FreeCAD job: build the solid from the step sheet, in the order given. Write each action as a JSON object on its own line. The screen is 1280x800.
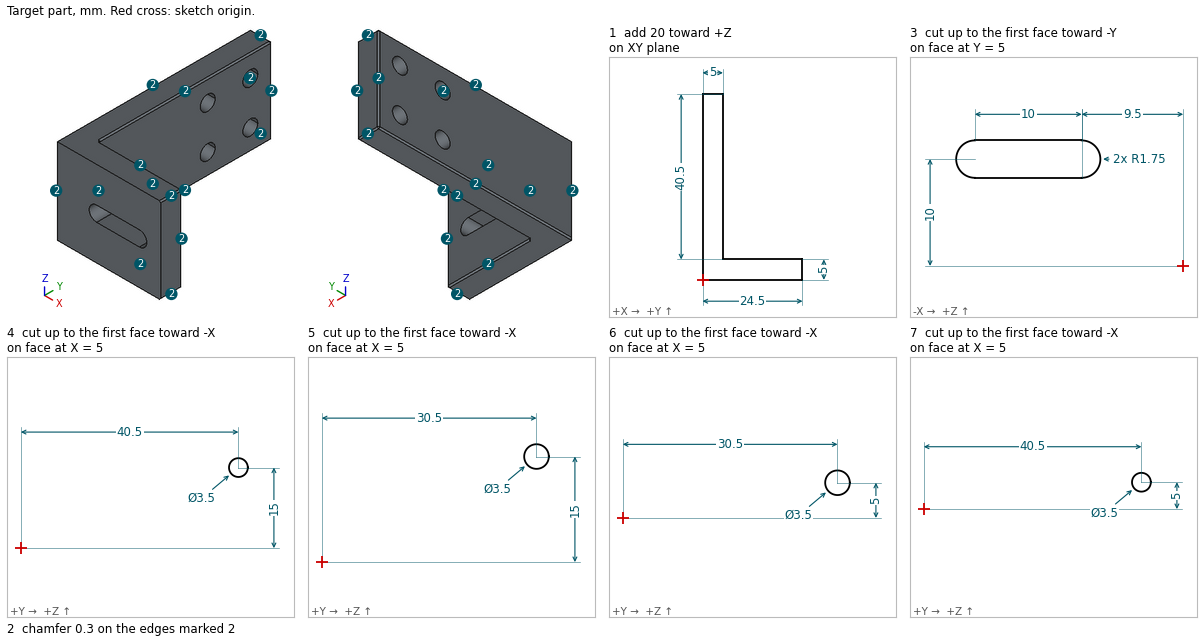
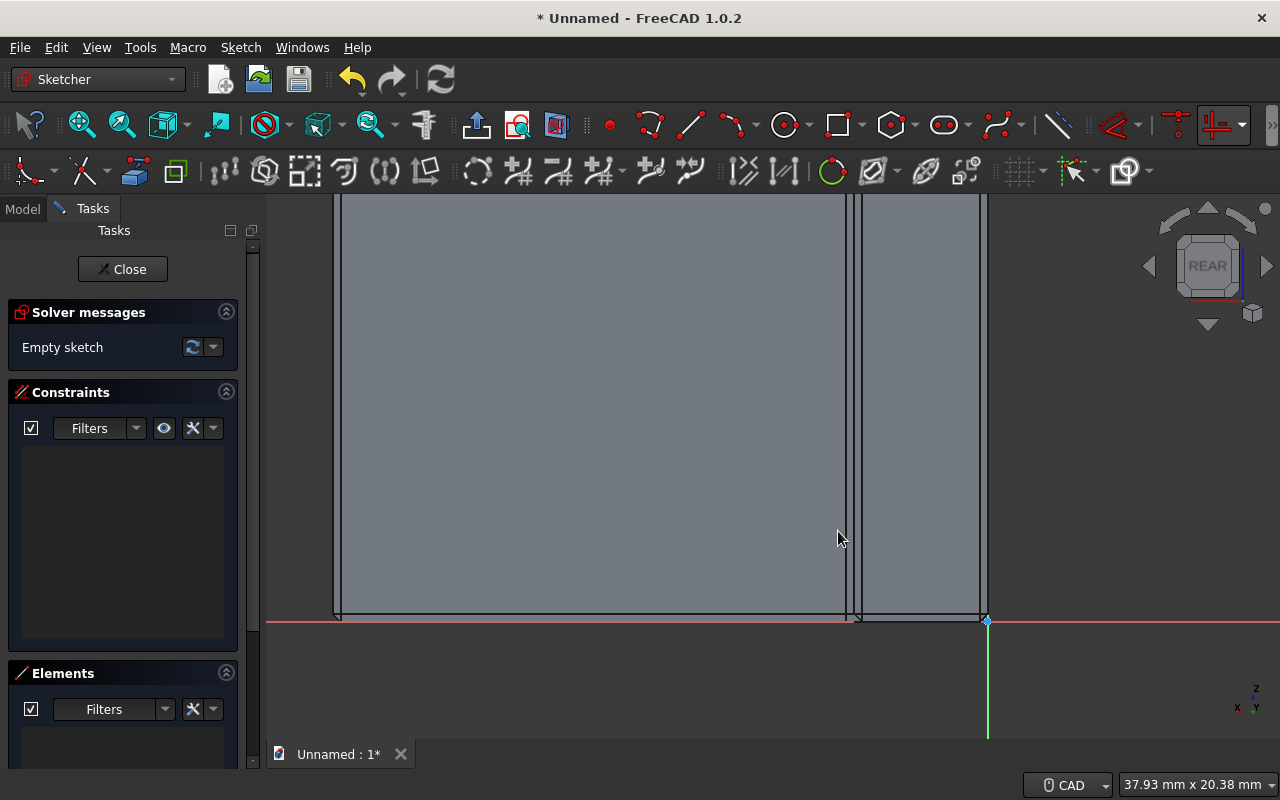
{"action": "left_click", "coordinate": [467, 355]}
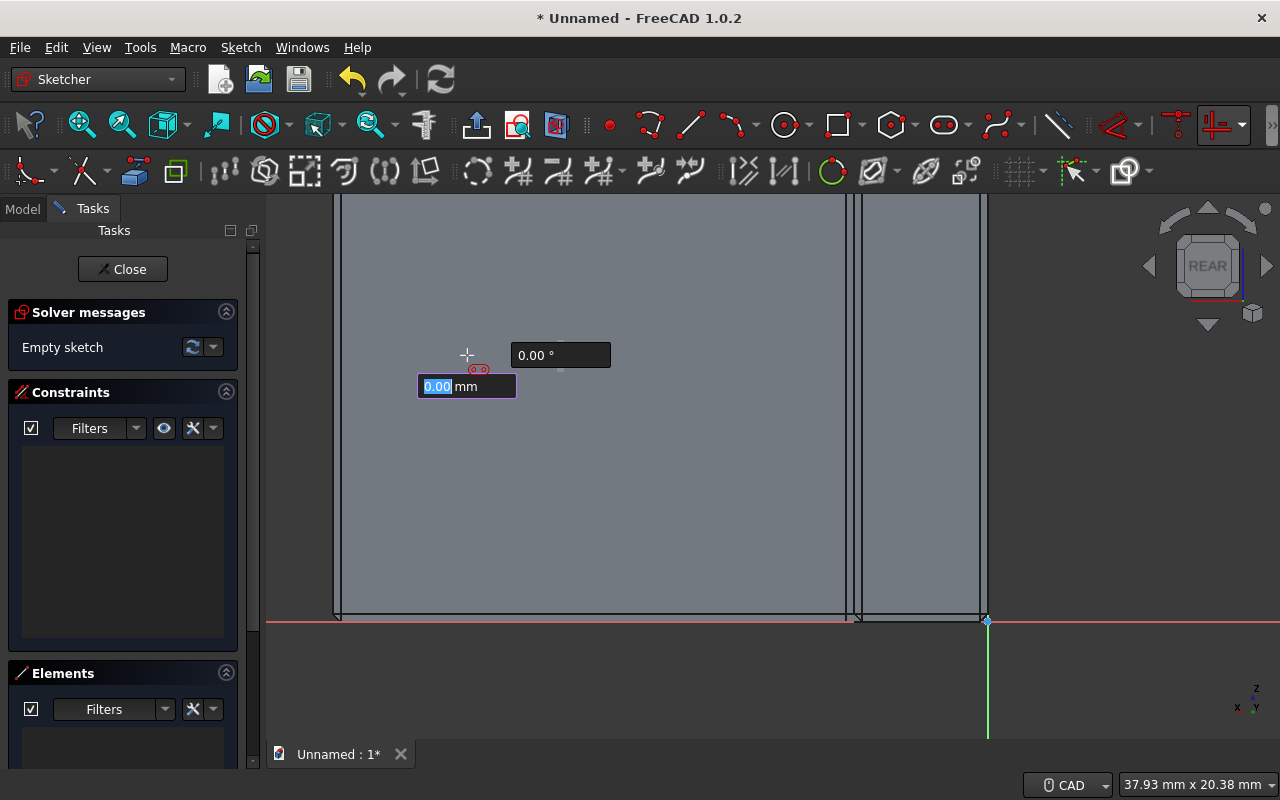
{"action": "left_click", "coordinate": [734, 355]}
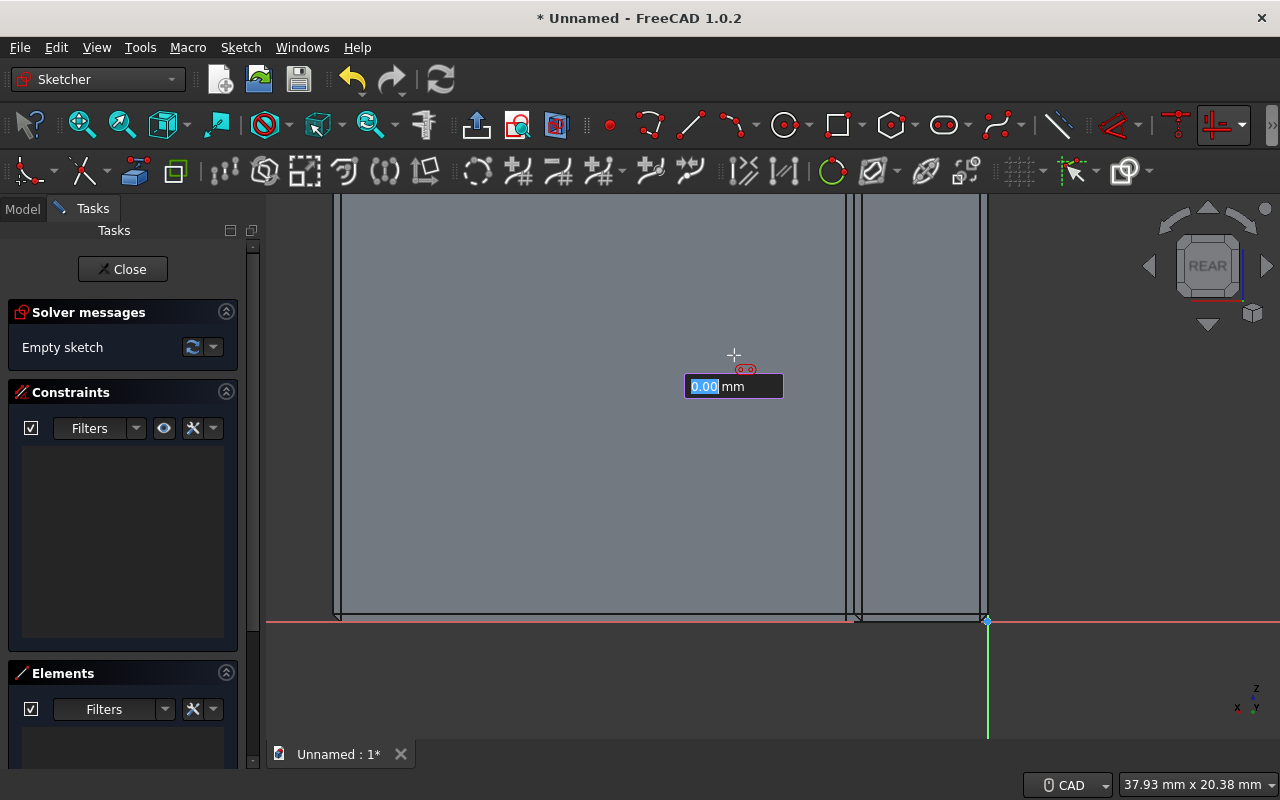
{"action": "left_click", "coordinate": [600, 401]}
{"action": "key", "text": "Escape"}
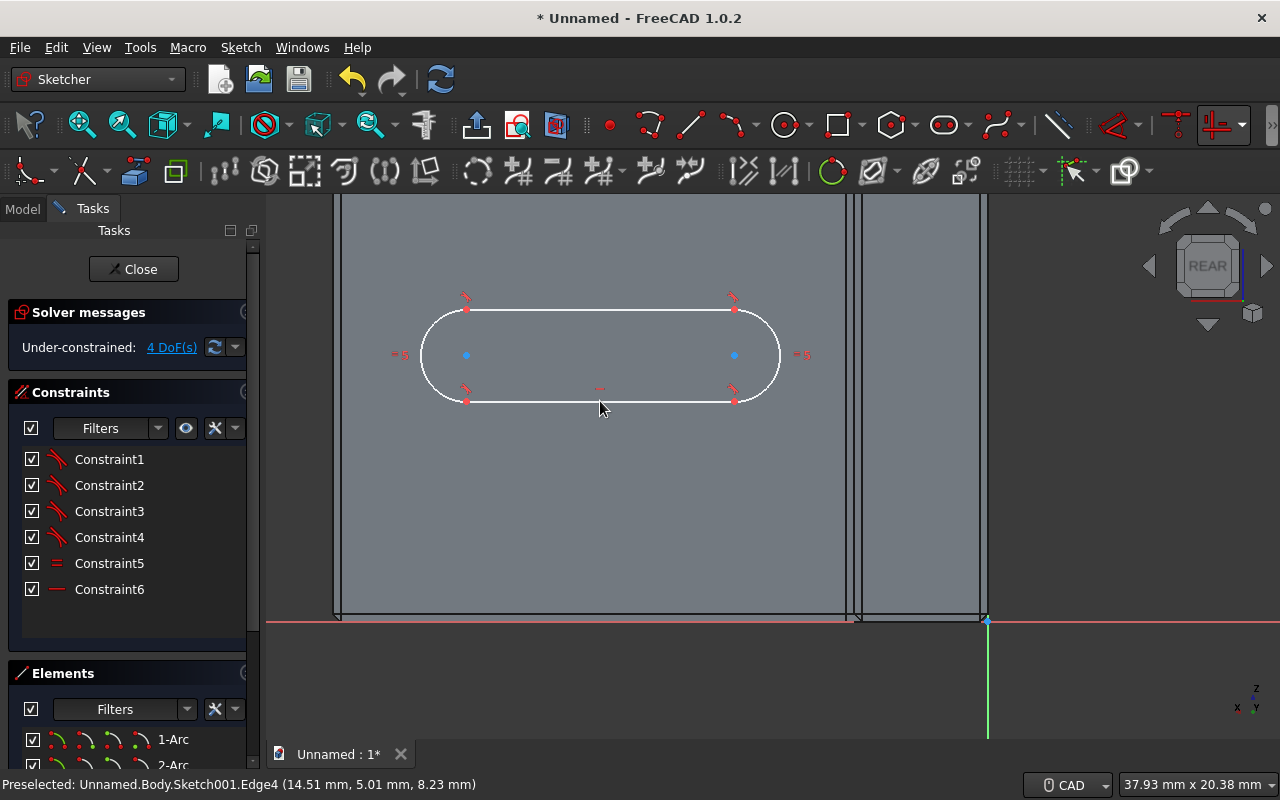
{"action": "left_click", "coordinate": [1114, 126]}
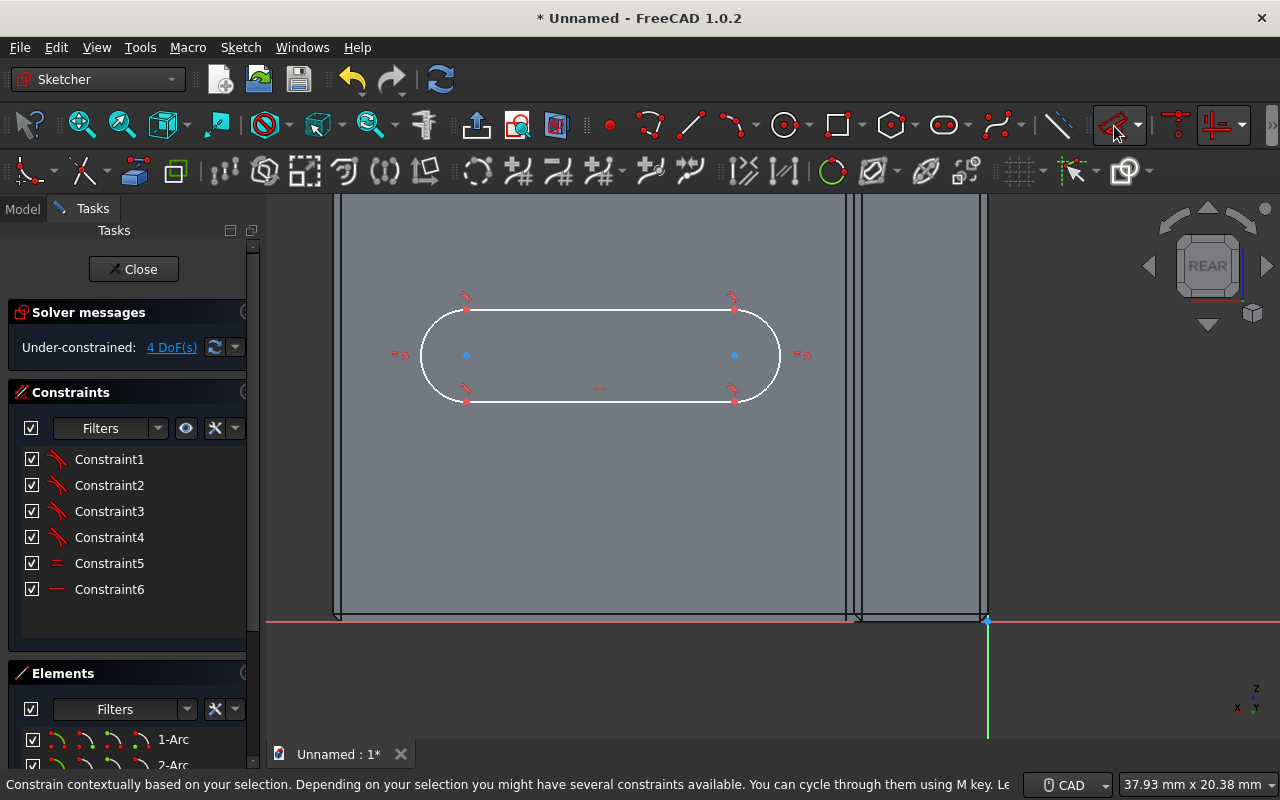
{"action": "left_click", "coordinate": [430, 329]}
{"action": "left_click", "coordinate": [404, 310]}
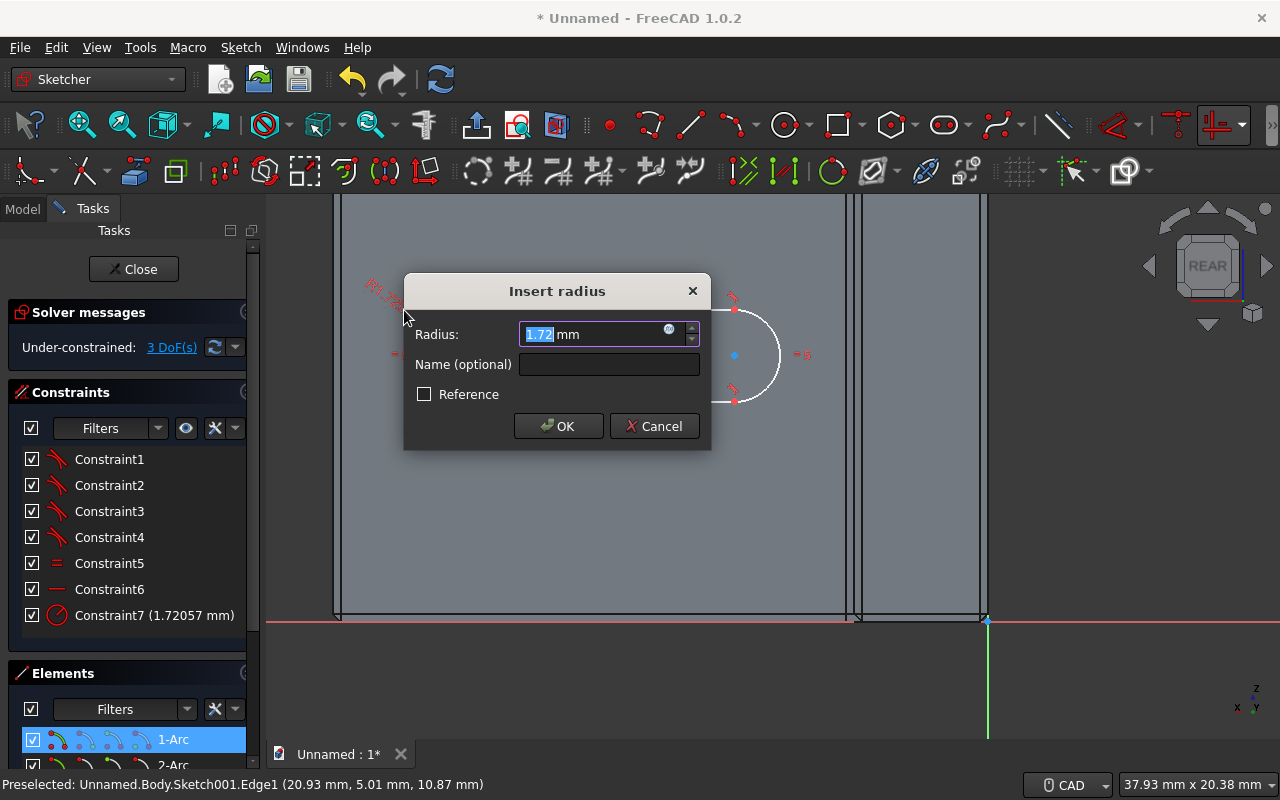
{"action": "type", "text": "1.75"}
{"action": "key", "text": "Return"}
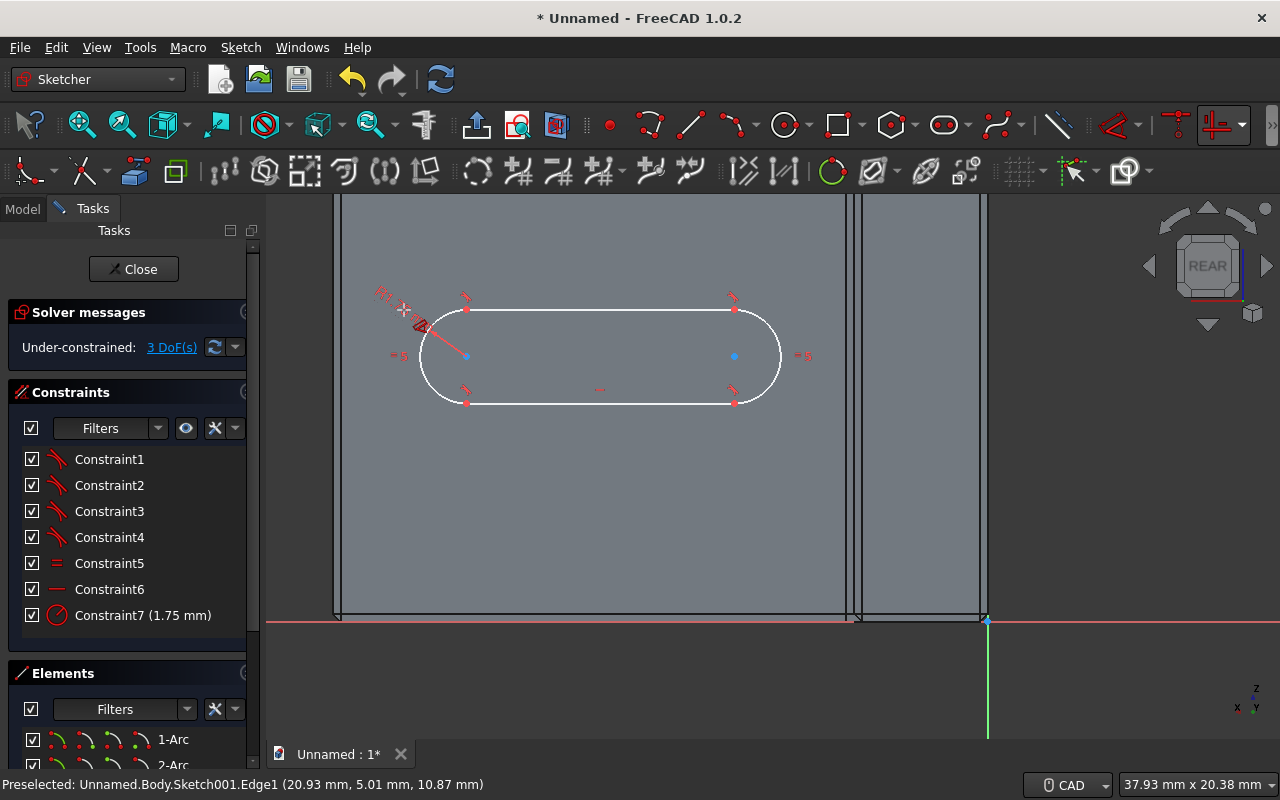
{"action": "left_click", "coordinate": [547, 310]}
{"action": "left_click", "coordinate": [601, 276]}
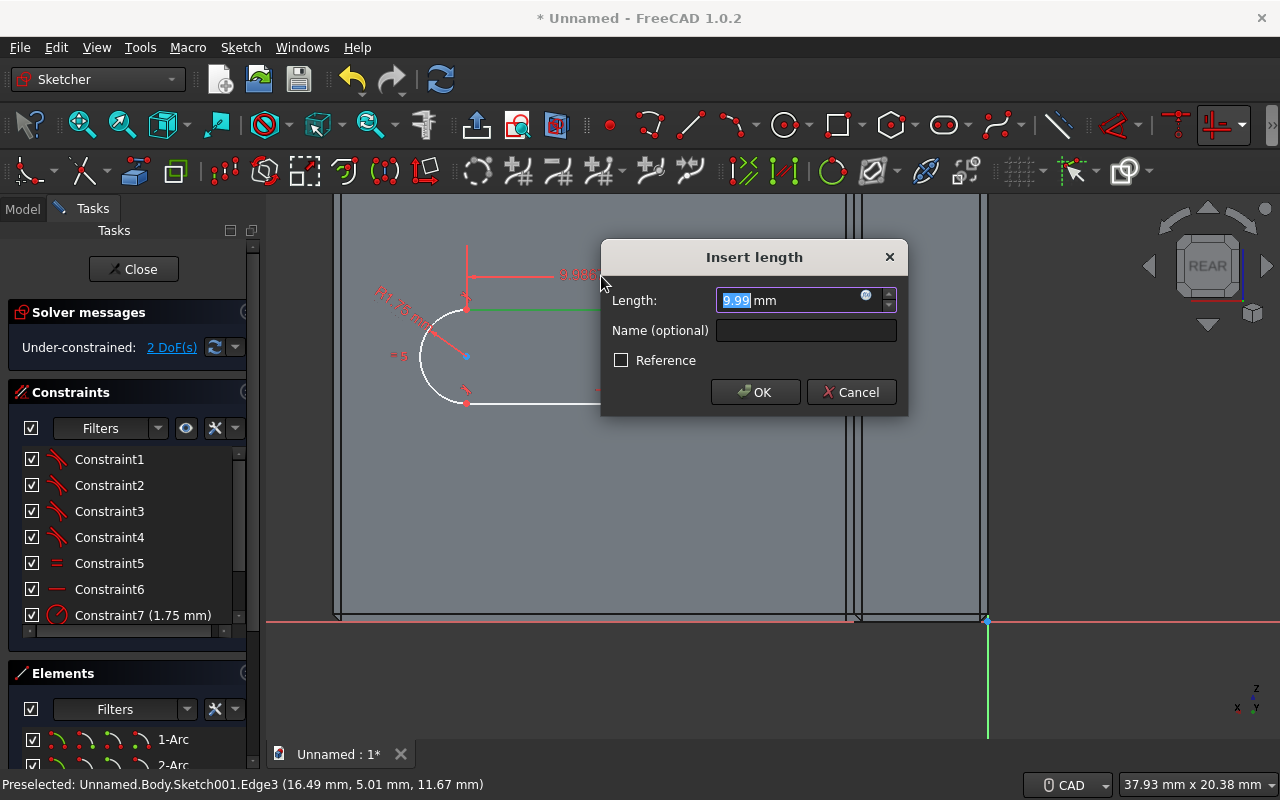
{"action": "type", "text": "10"}
{"action": "key", "text": "Return"}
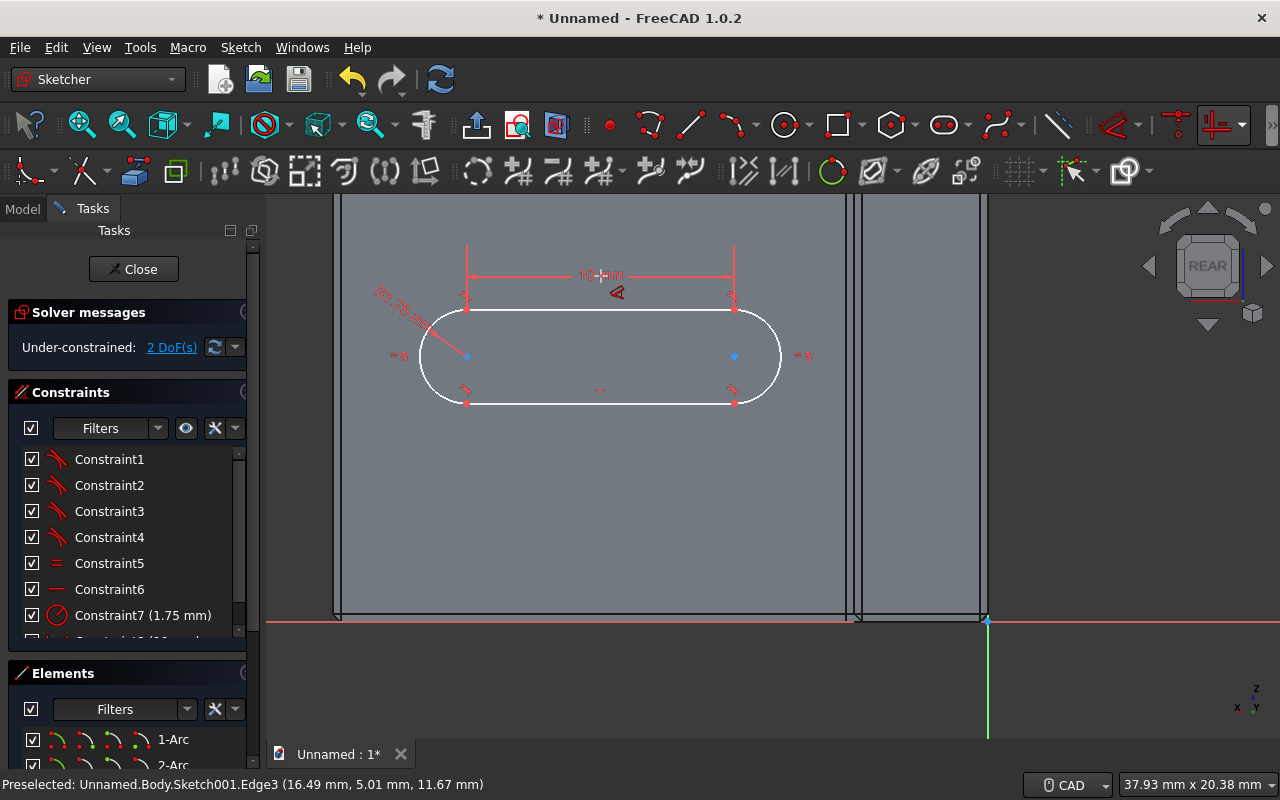
{"action": "left_click", "coordinate": [467, 357]}
{"action": "left_click", "coordinate": [1022, 489]}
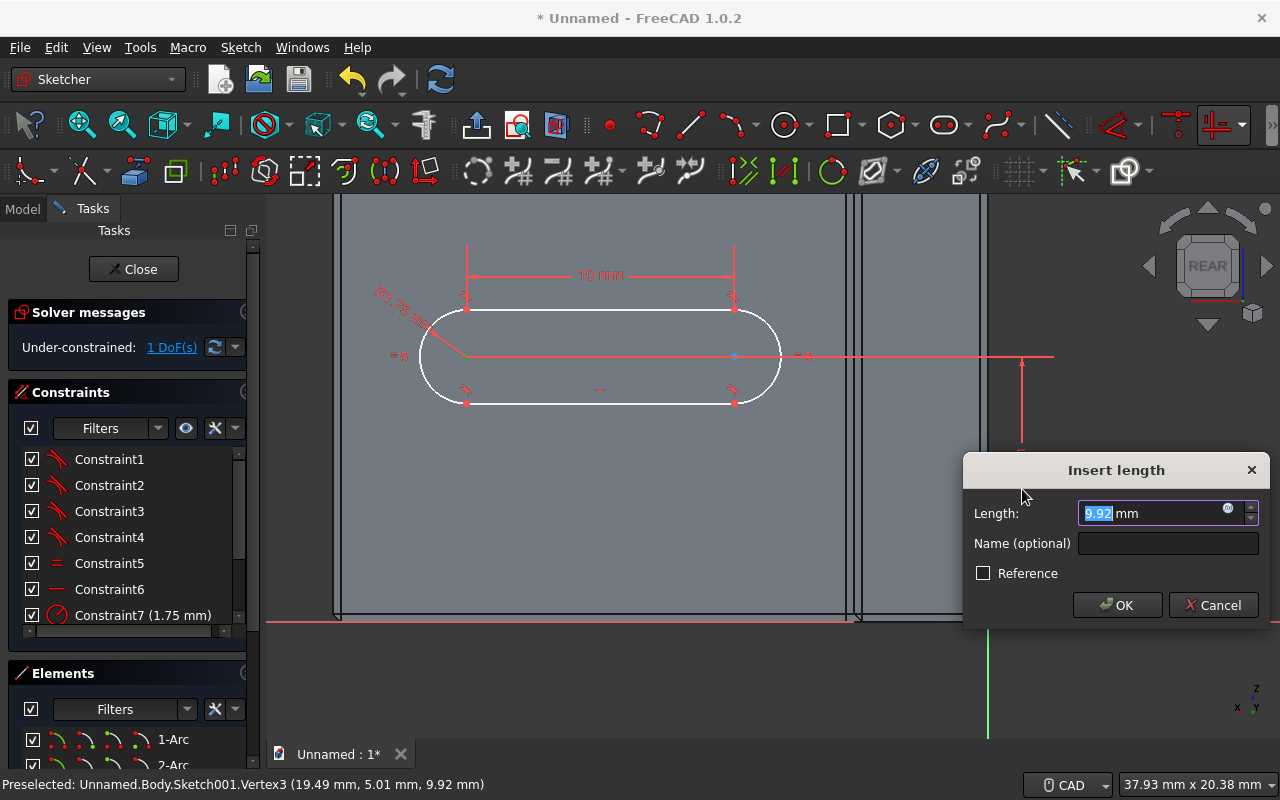
{"action": "type", "text": "10"}
{"action": "key", "text": "Return"}